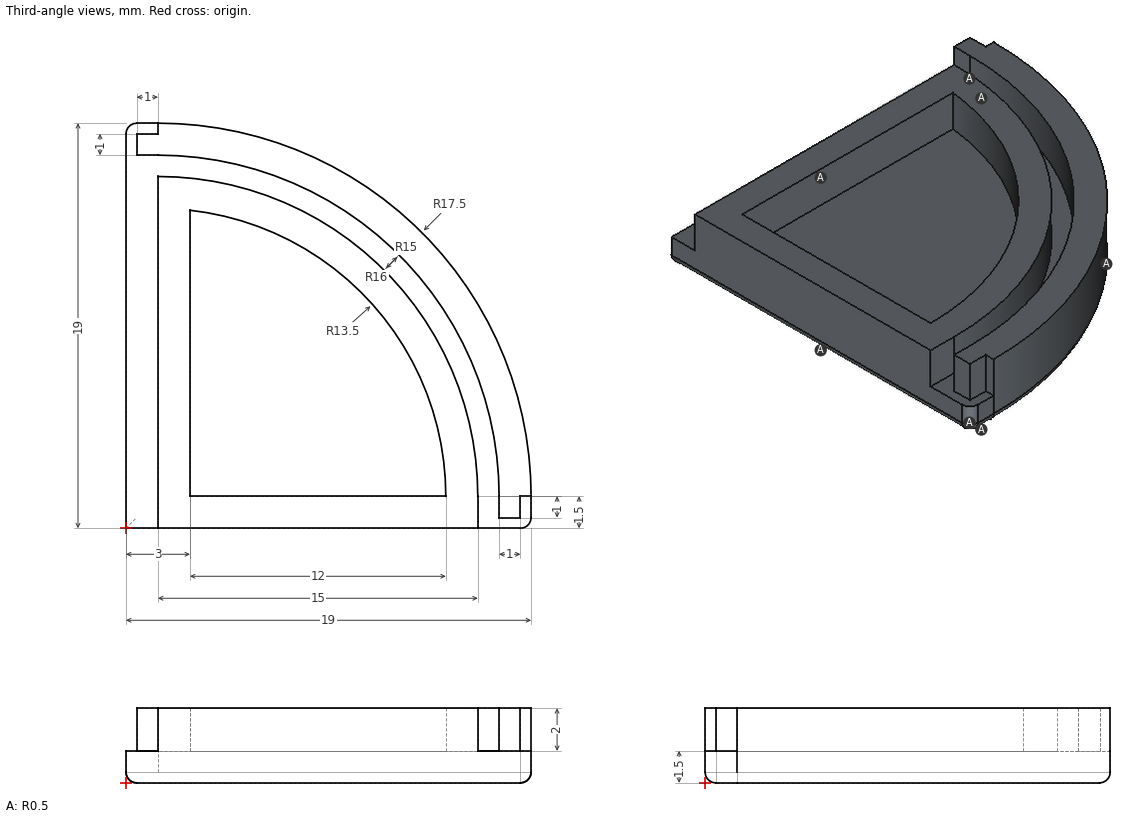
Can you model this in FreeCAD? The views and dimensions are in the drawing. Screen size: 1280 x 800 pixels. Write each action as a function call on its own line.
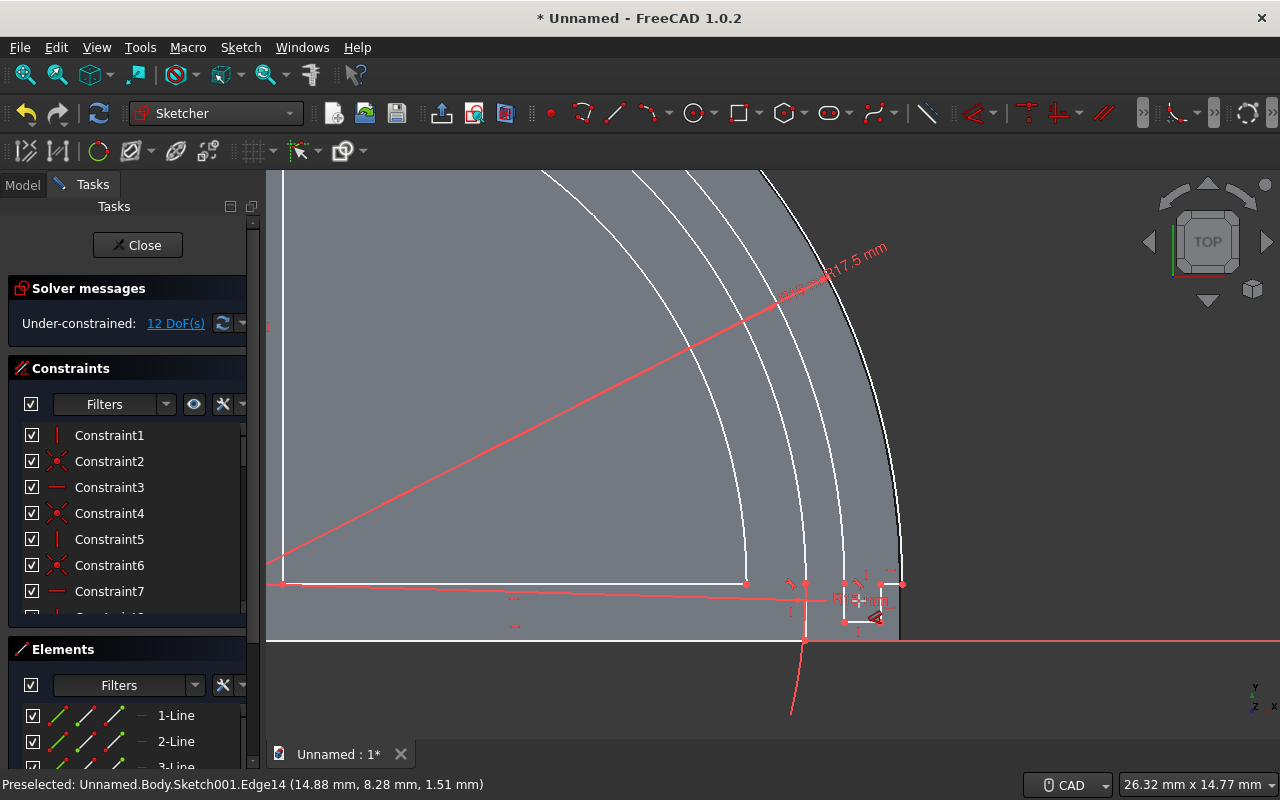
click(698, 363)
click(727, 349)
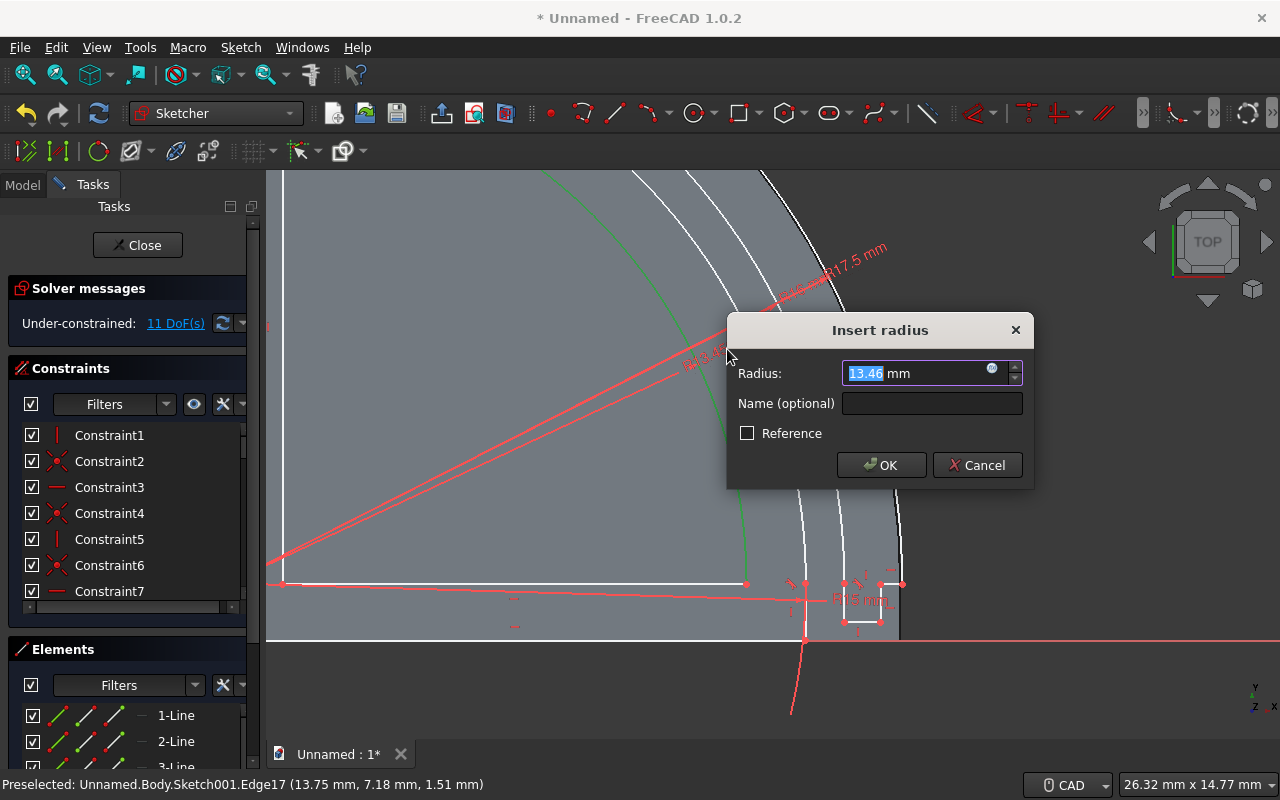
text(13.5)
key(Return)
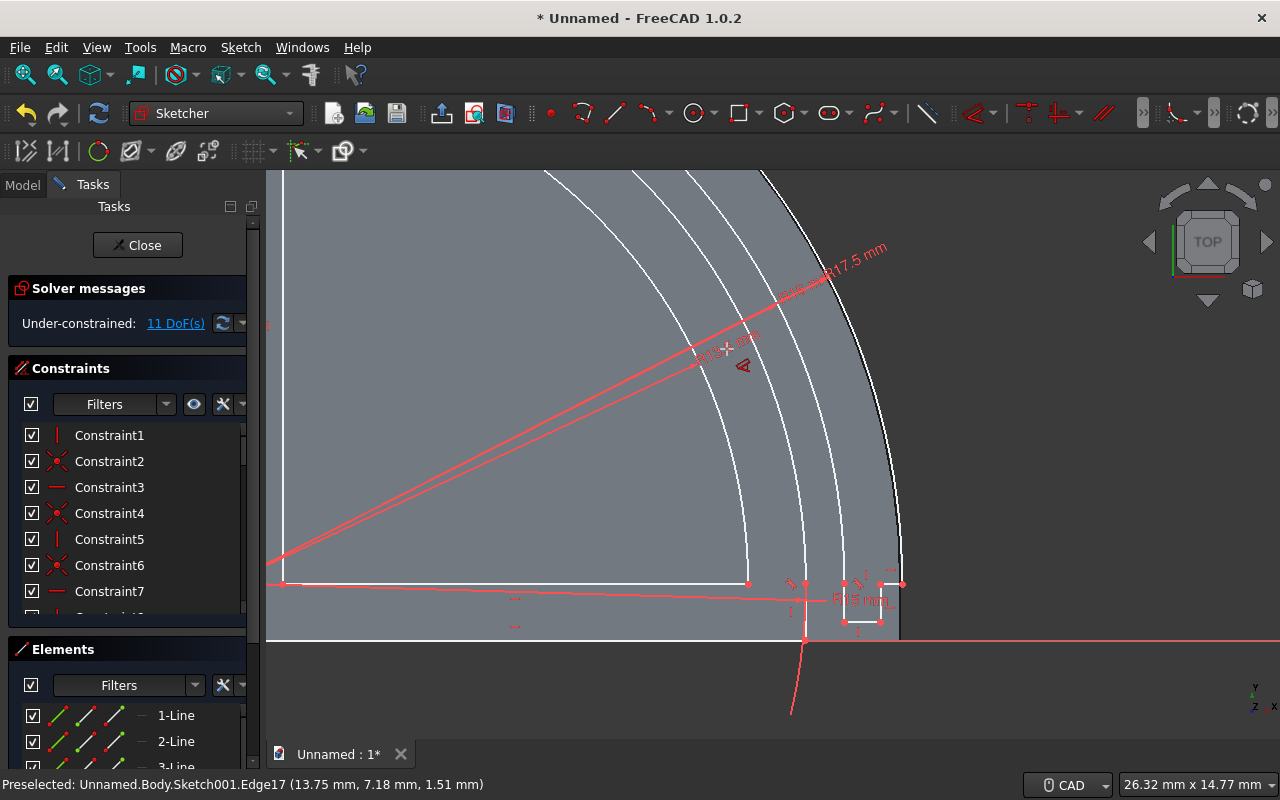
scroll(843, 601, down, 4)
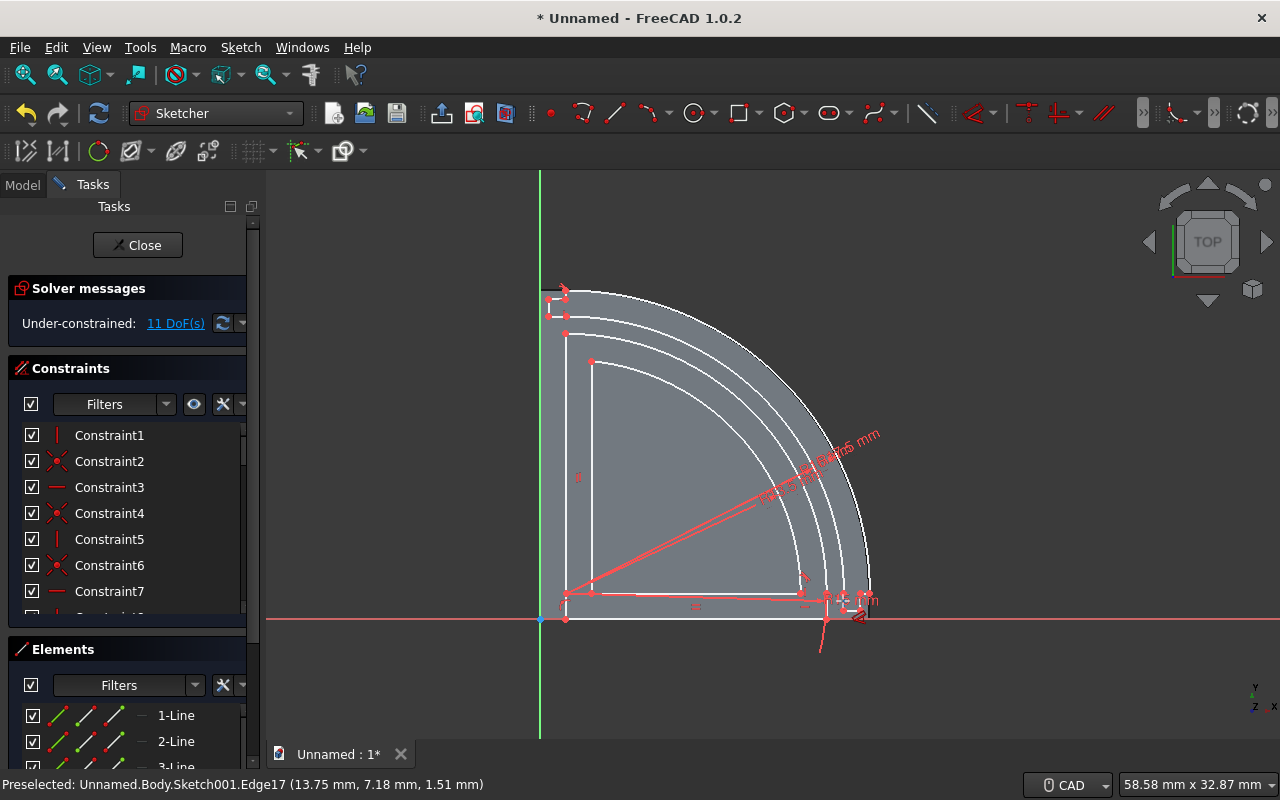
scroll(561, 299, up, 6)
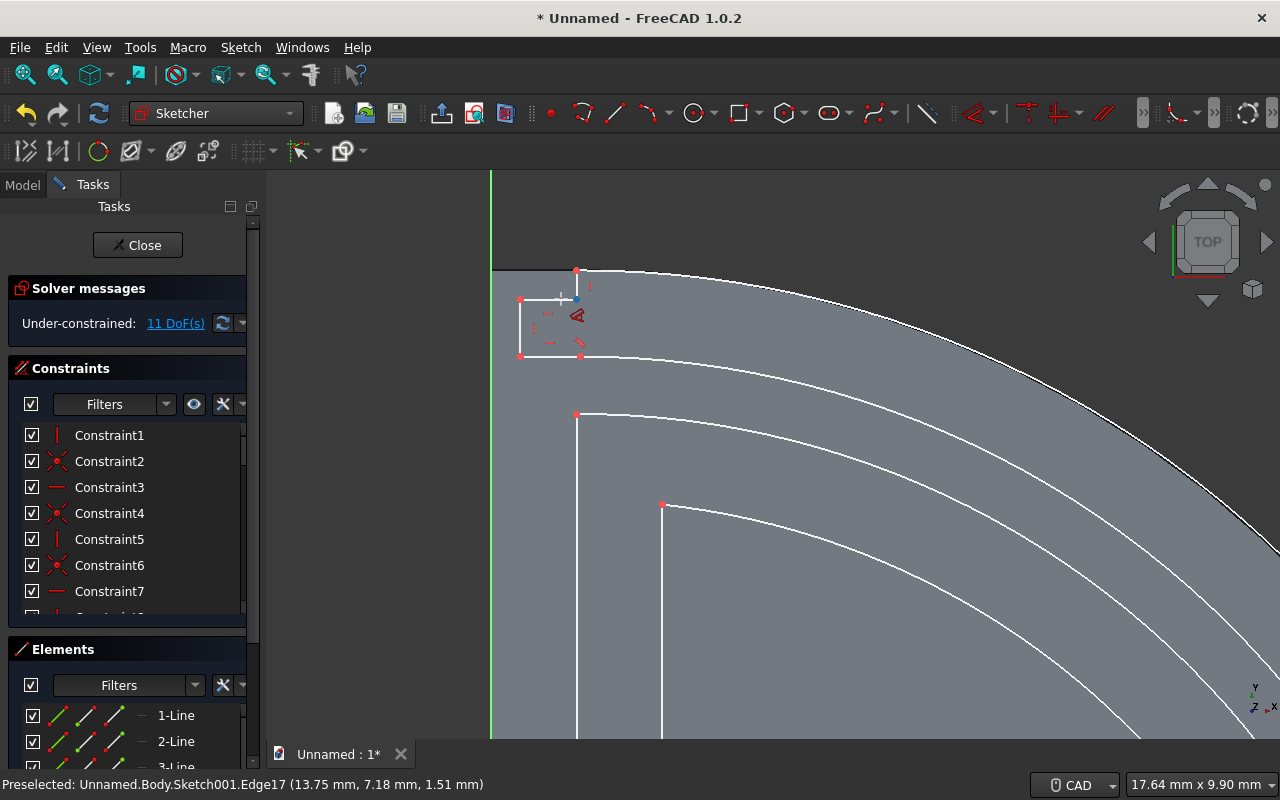
click(560, 300)
click(549, 266)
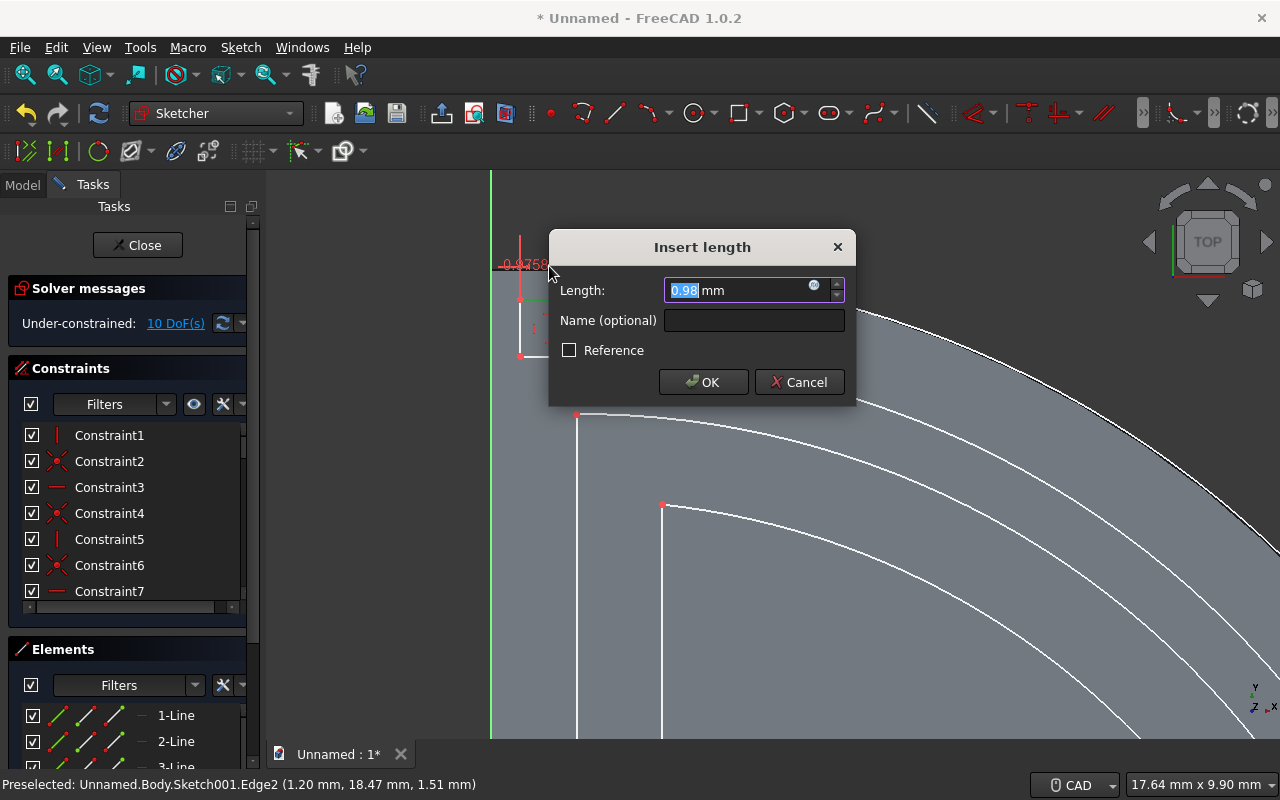
text(1)
key(Return)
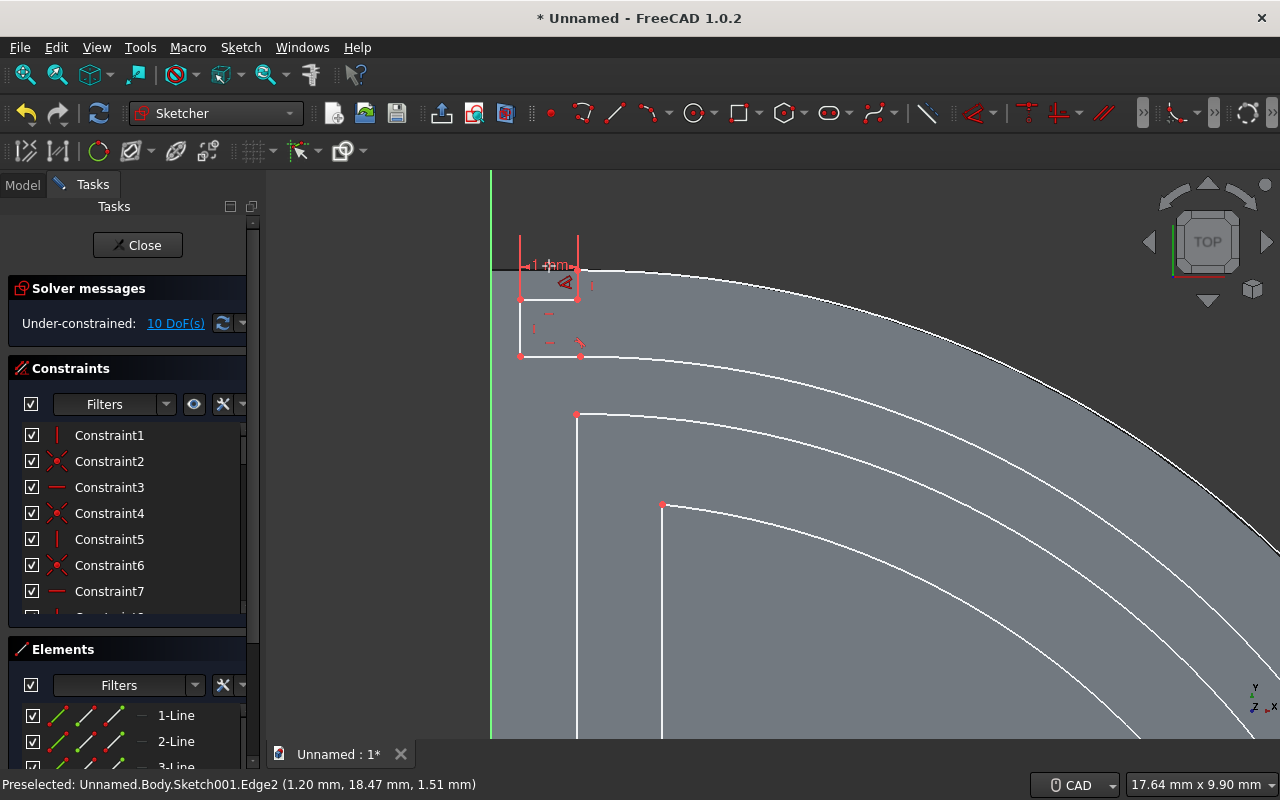
click(520, 317)
click(554, 328)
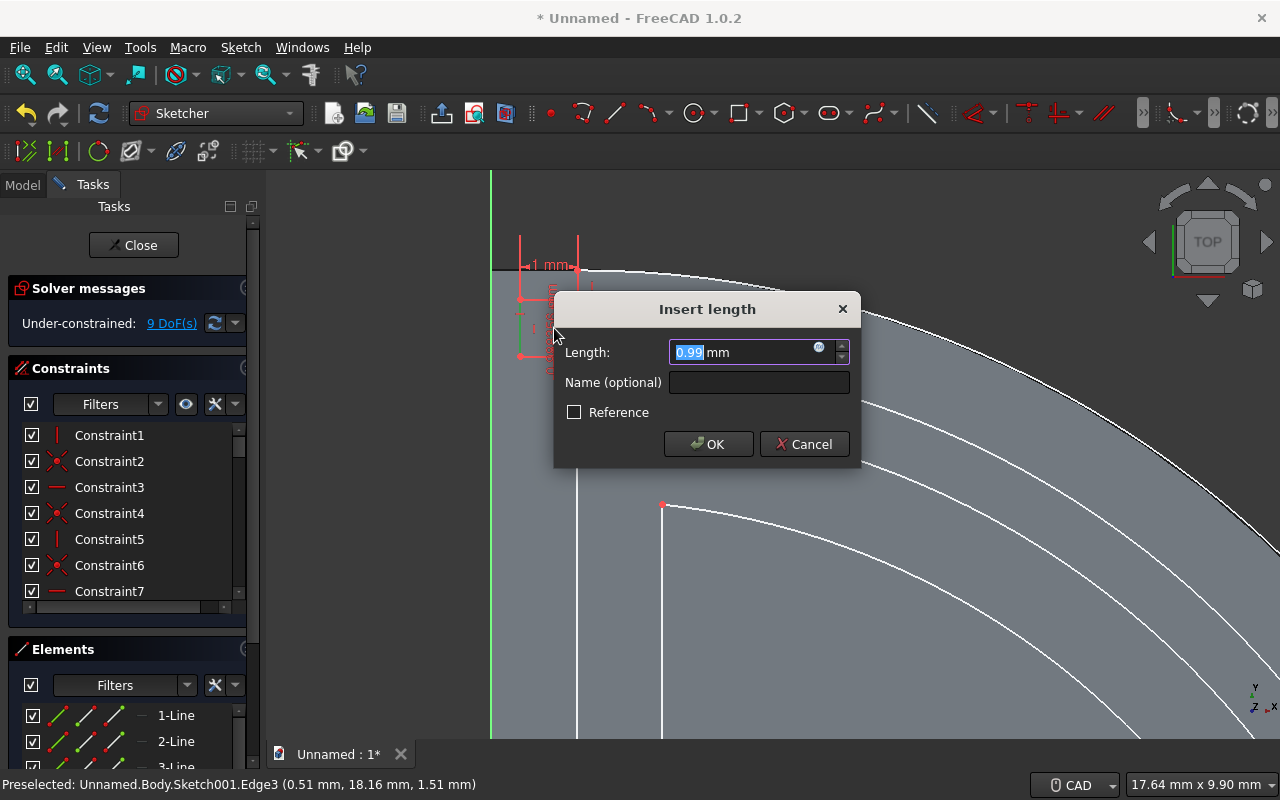
text(1)
key(Return)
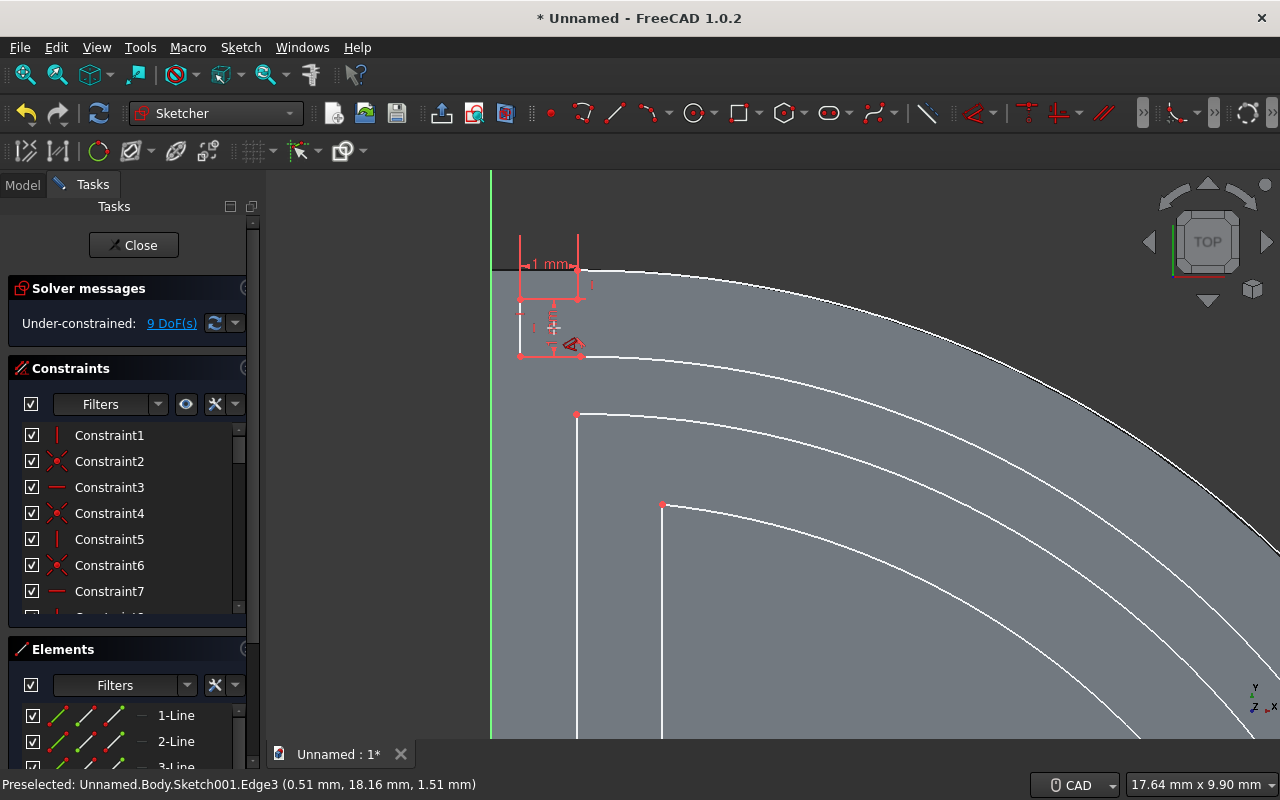
click(538, 357)
click(550, 391)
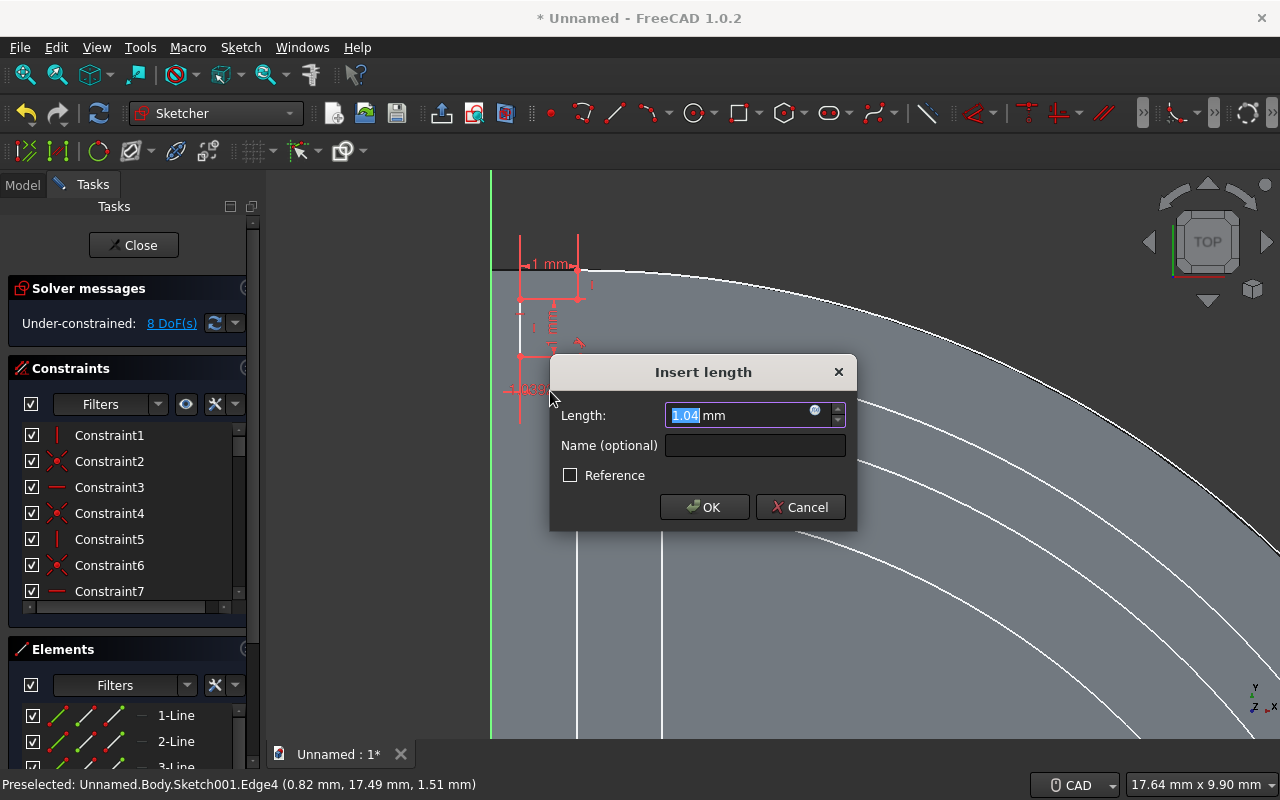
text(1)
key(Return)